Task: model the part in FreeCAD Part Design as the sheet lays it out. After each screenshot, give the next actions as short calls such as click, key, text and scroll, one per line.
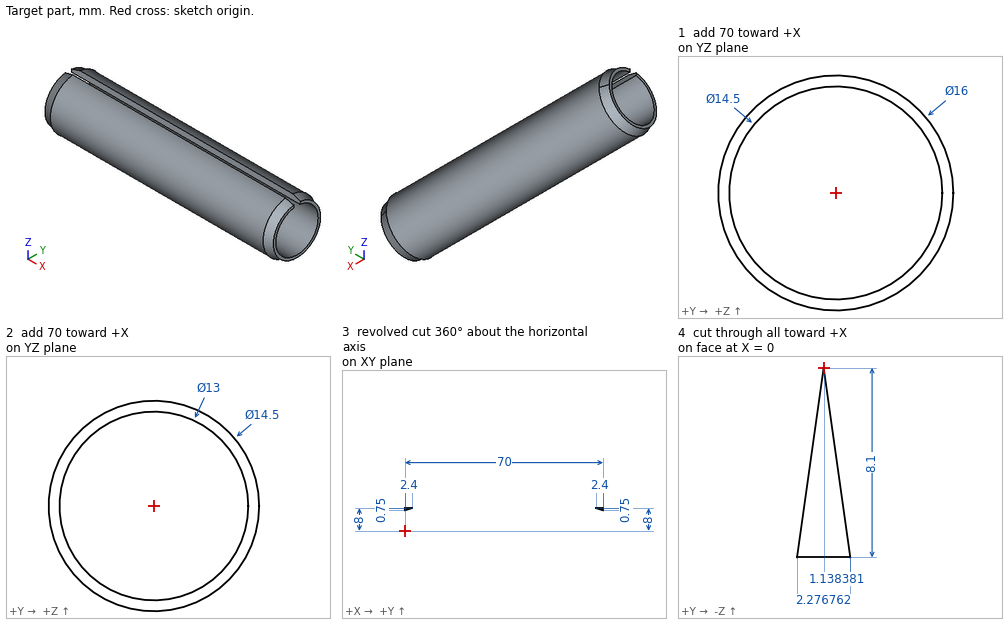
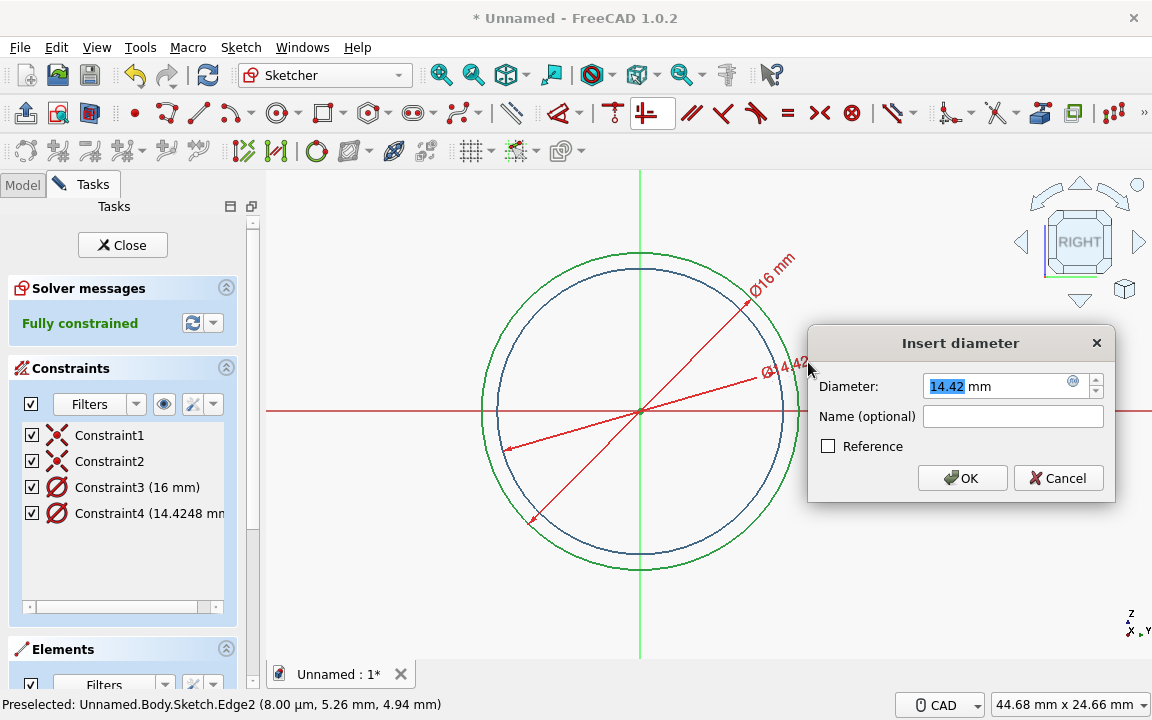
text(14.5)
key(Return)
key(Escape)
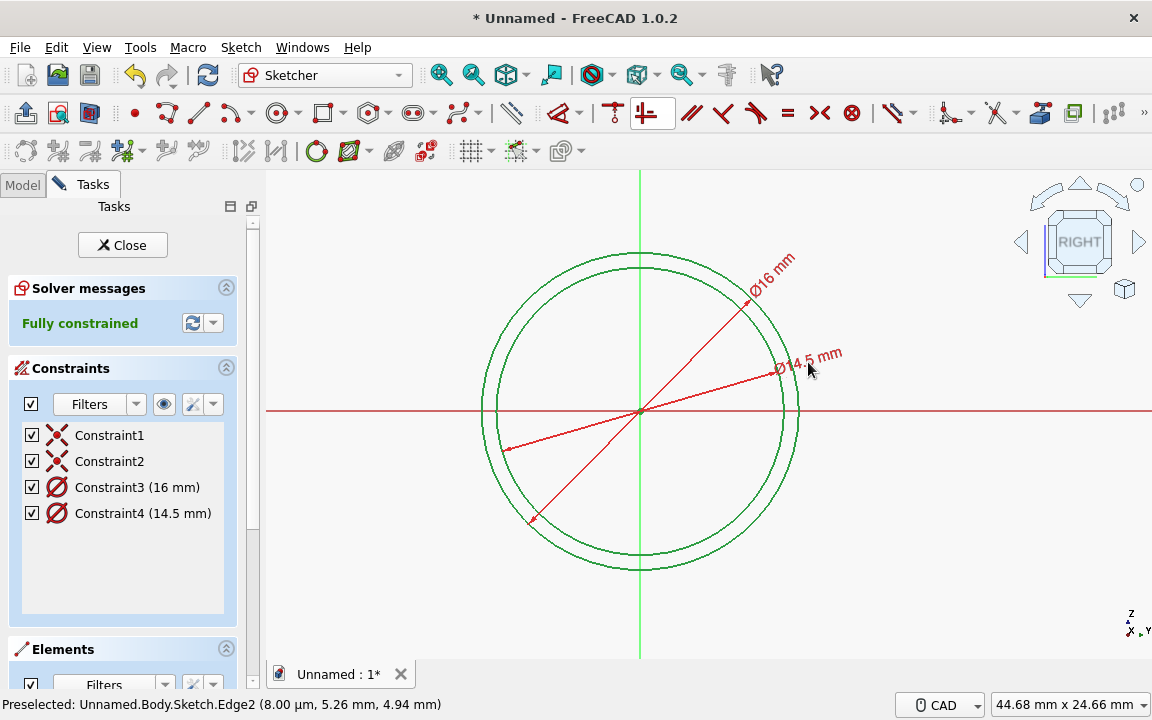
click(123, 245)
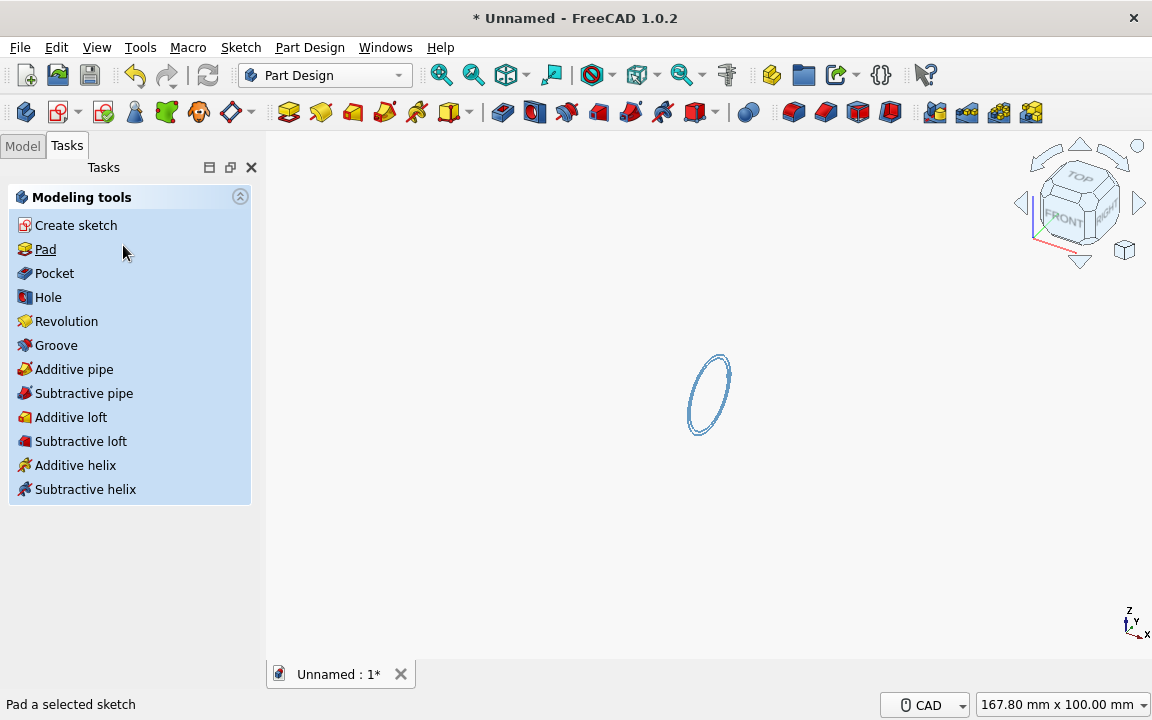
click(290, 112)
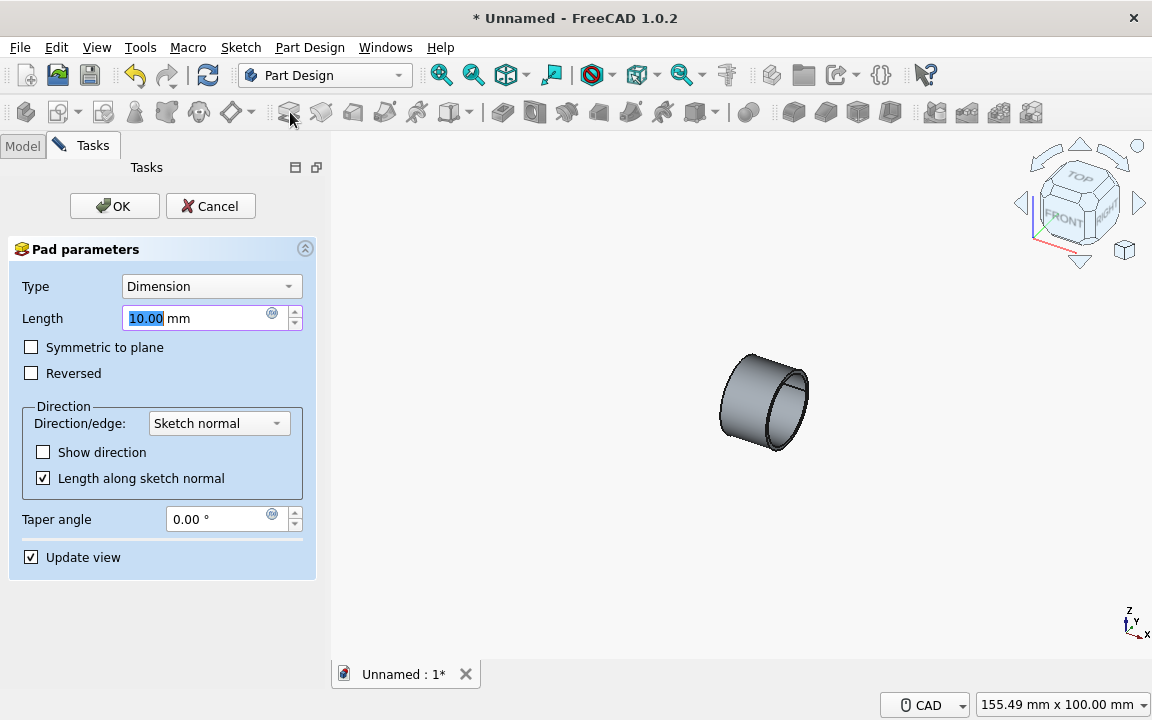
text(70)
key(Tab)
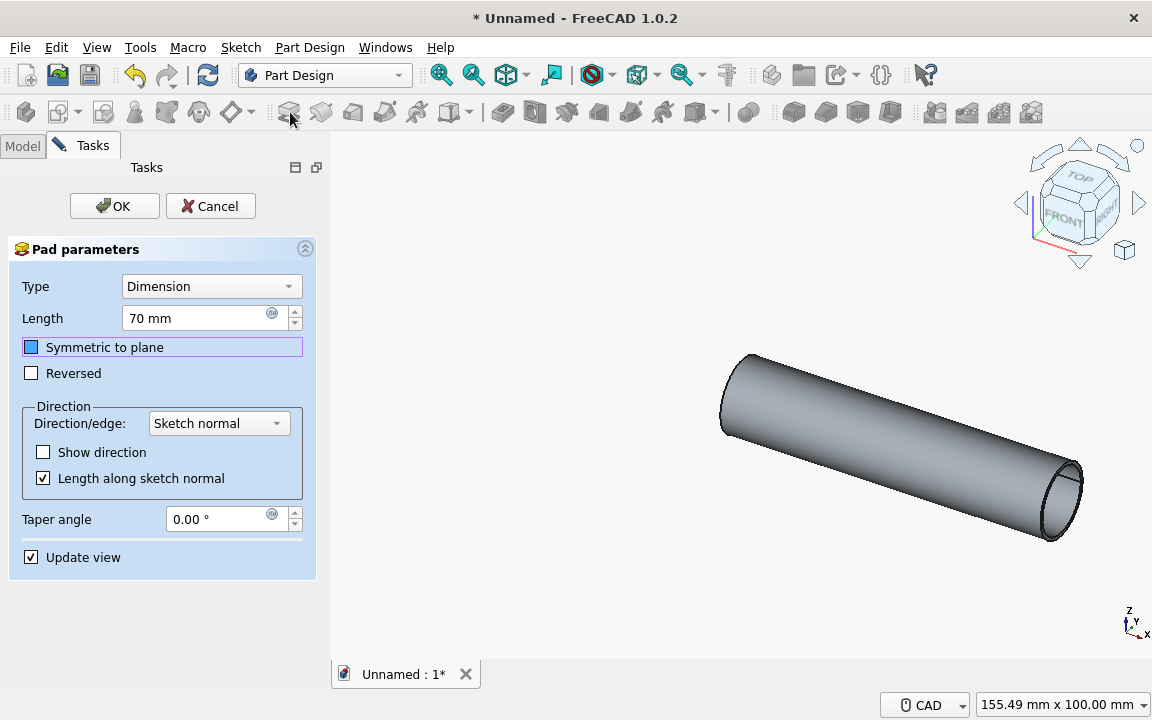
click(115, 206)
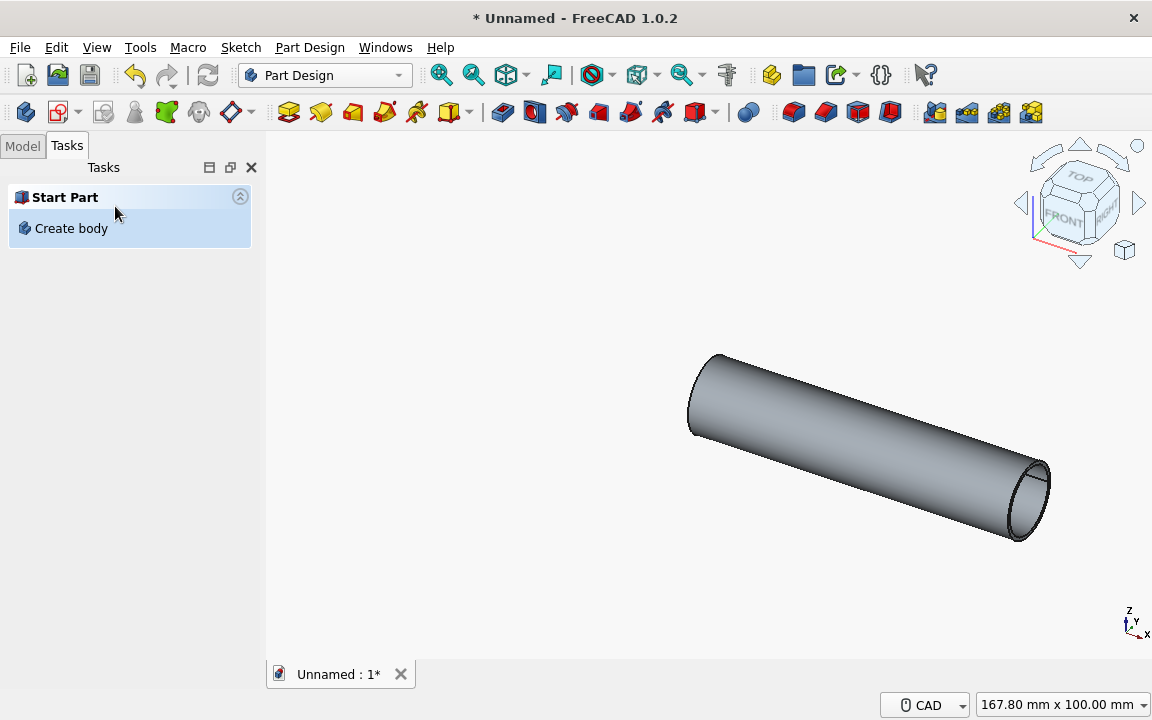
click(442, 76)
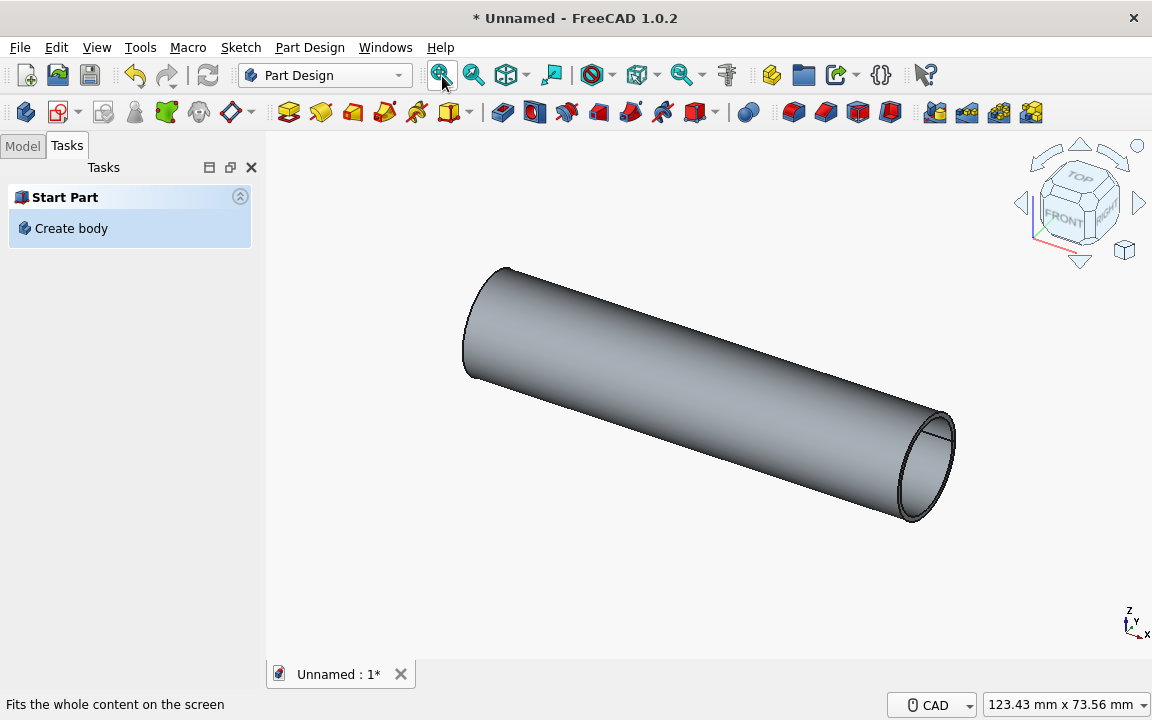
click(58, 112)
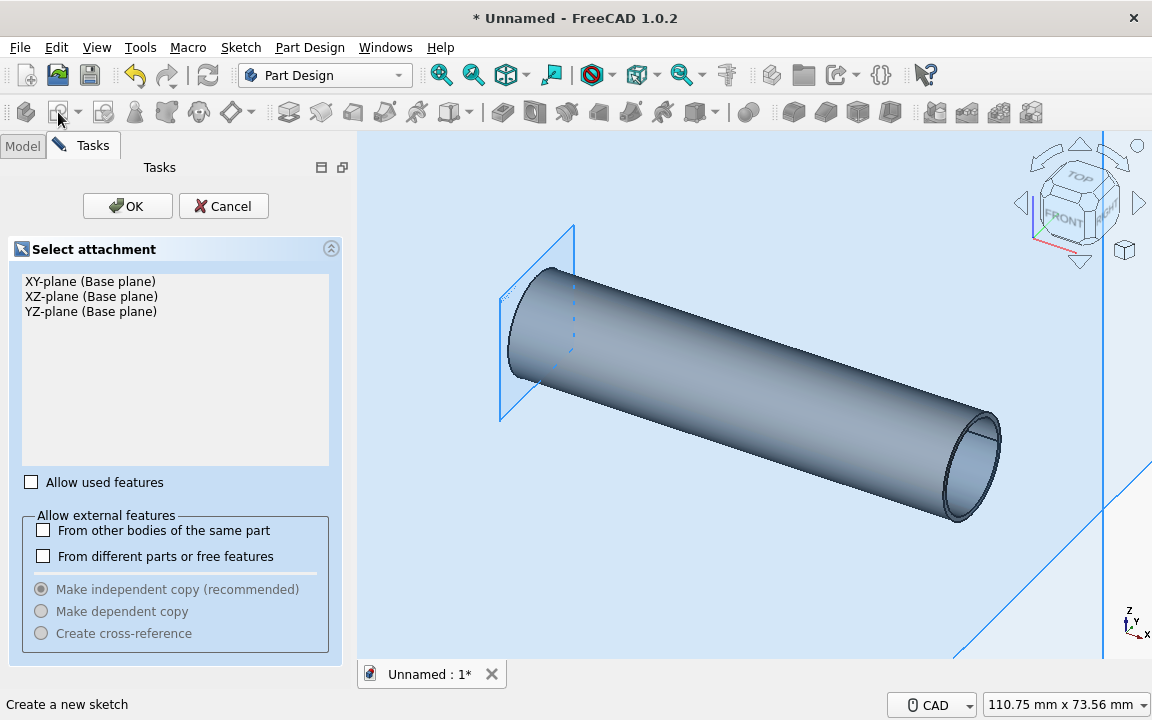
click(82, 312)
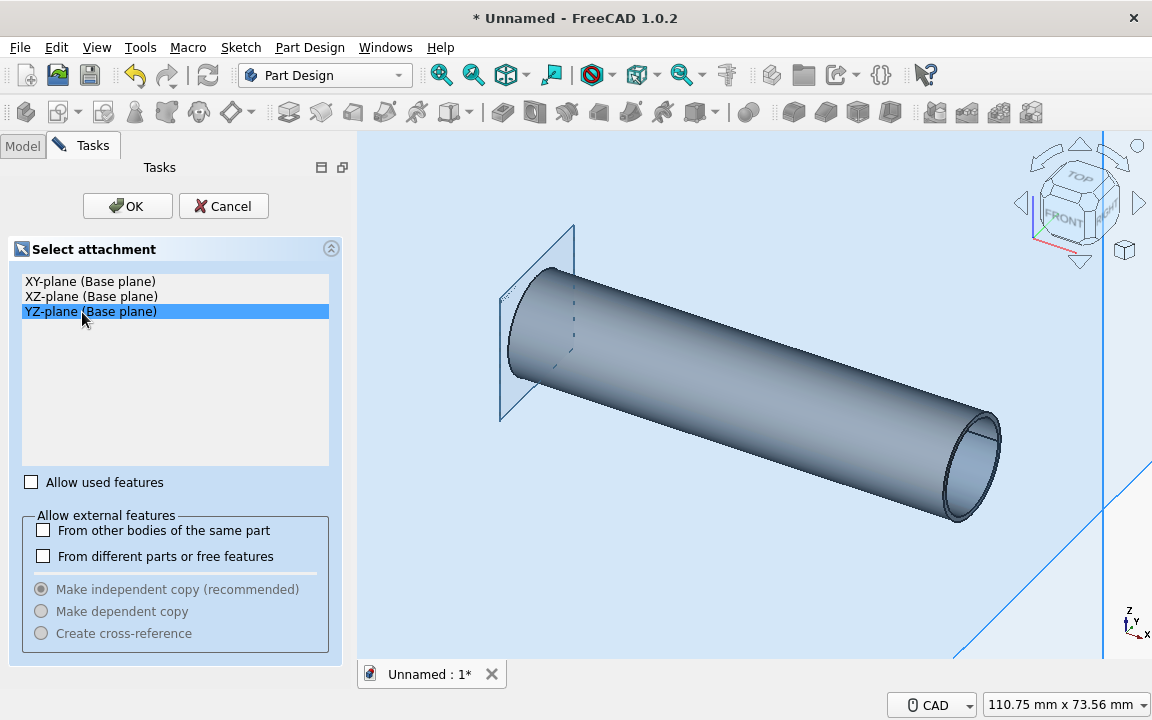
click(128, 206)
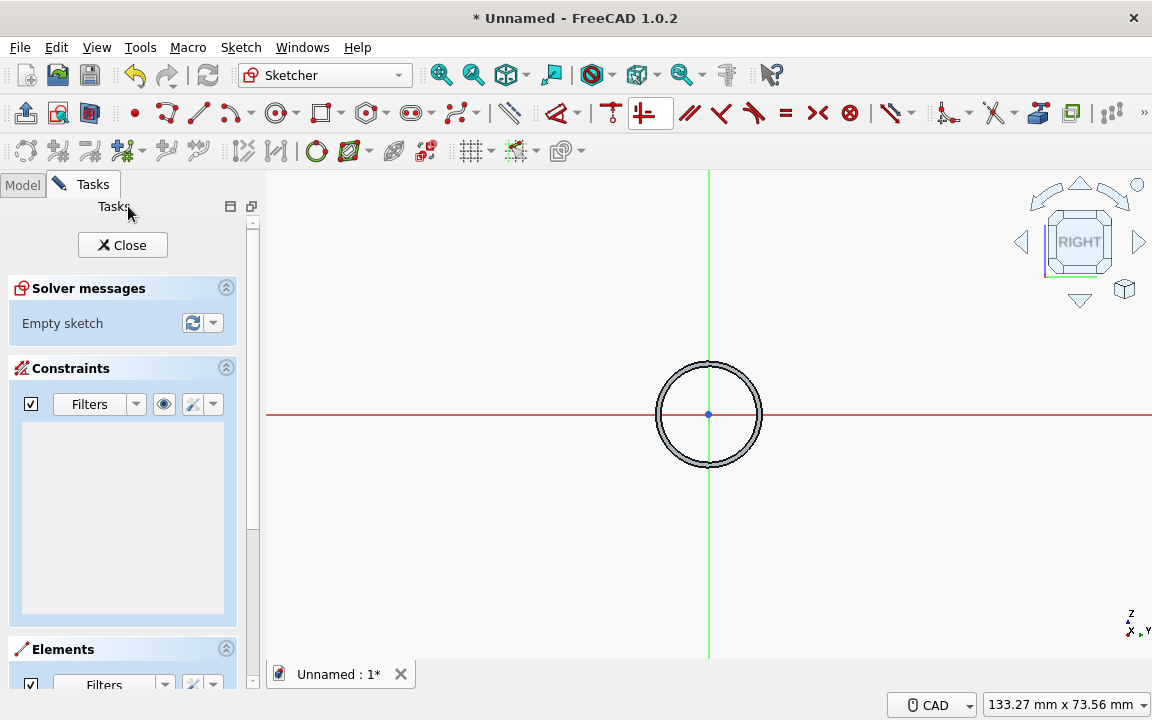
key(q)
key(s)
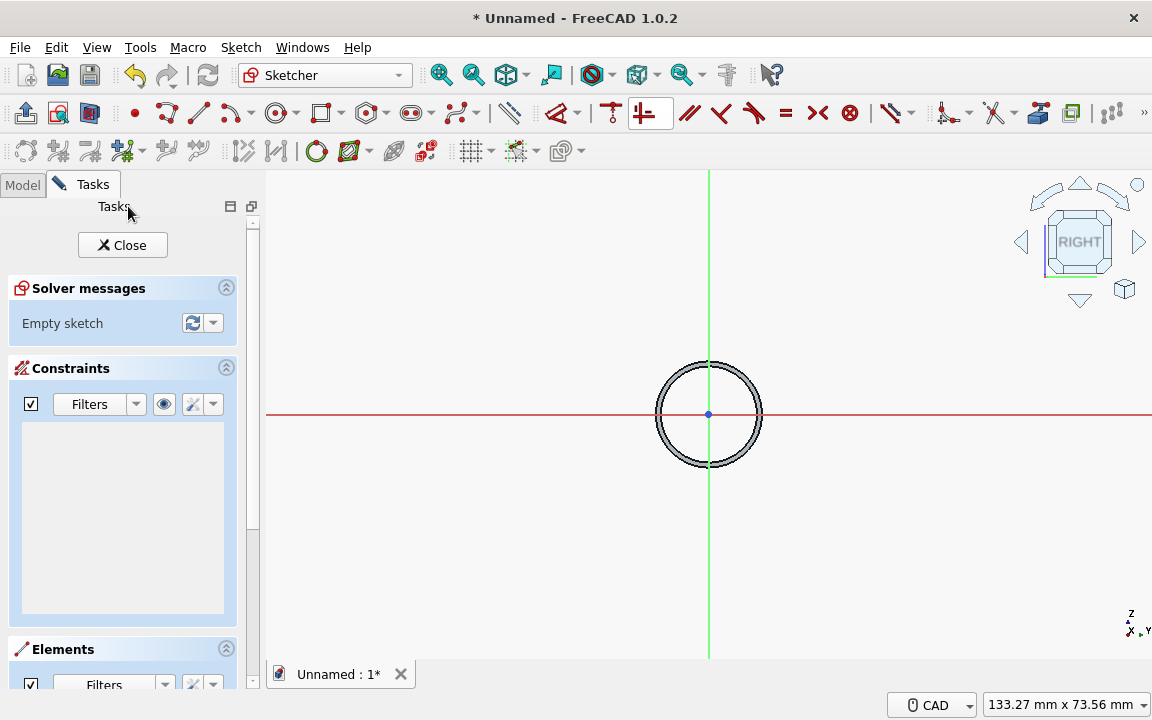
scroll(738, 415, up, 6)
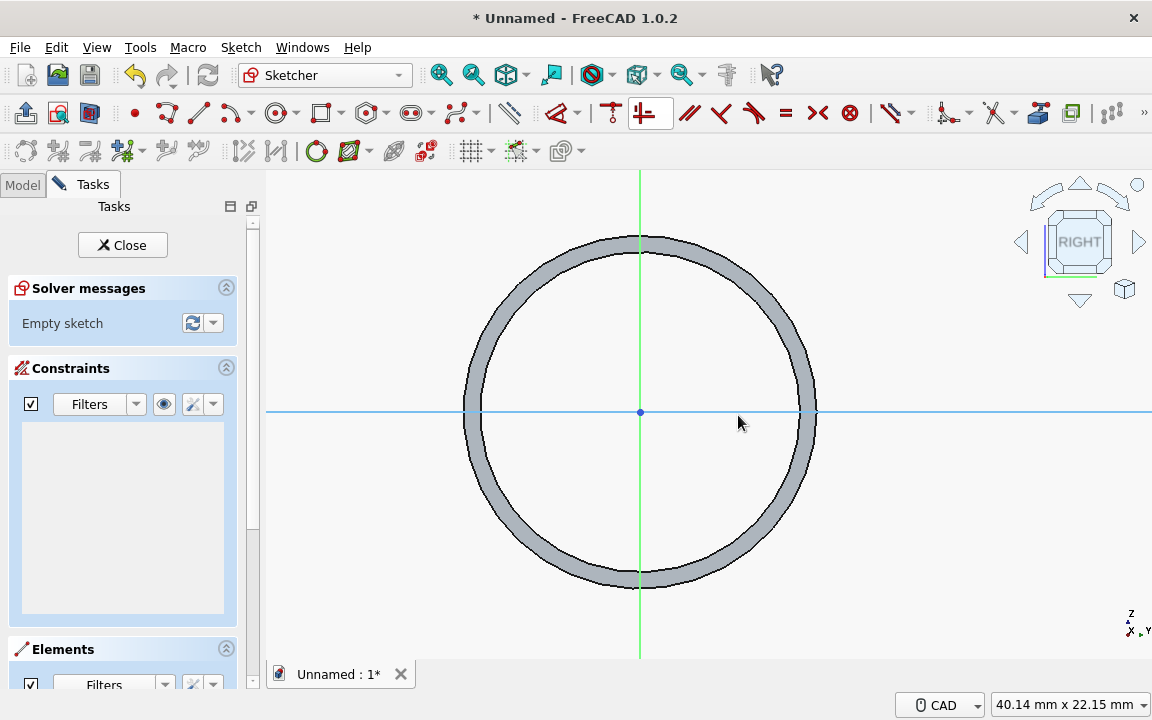
click(276, 114)